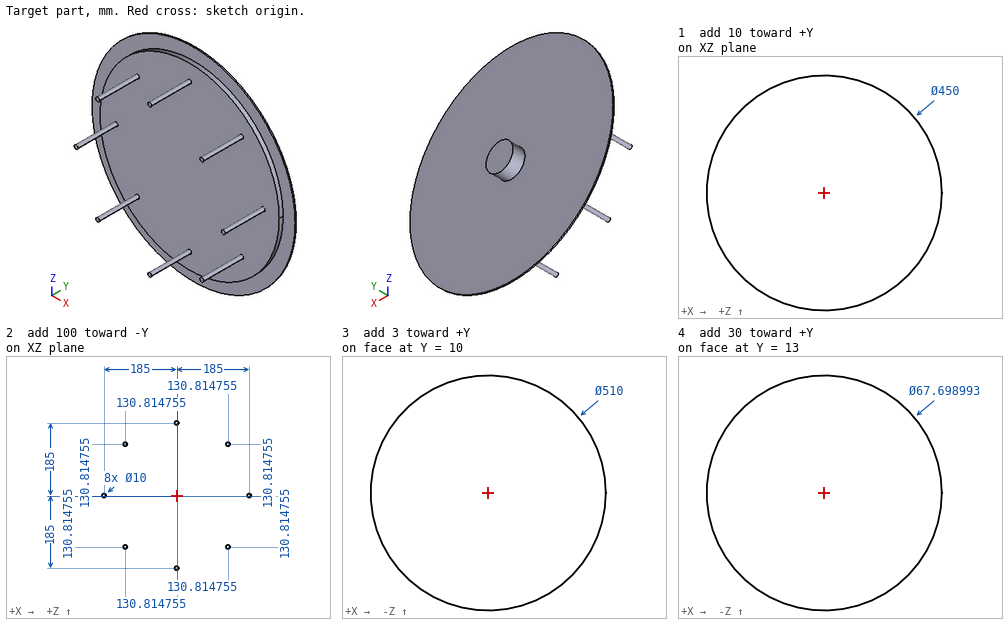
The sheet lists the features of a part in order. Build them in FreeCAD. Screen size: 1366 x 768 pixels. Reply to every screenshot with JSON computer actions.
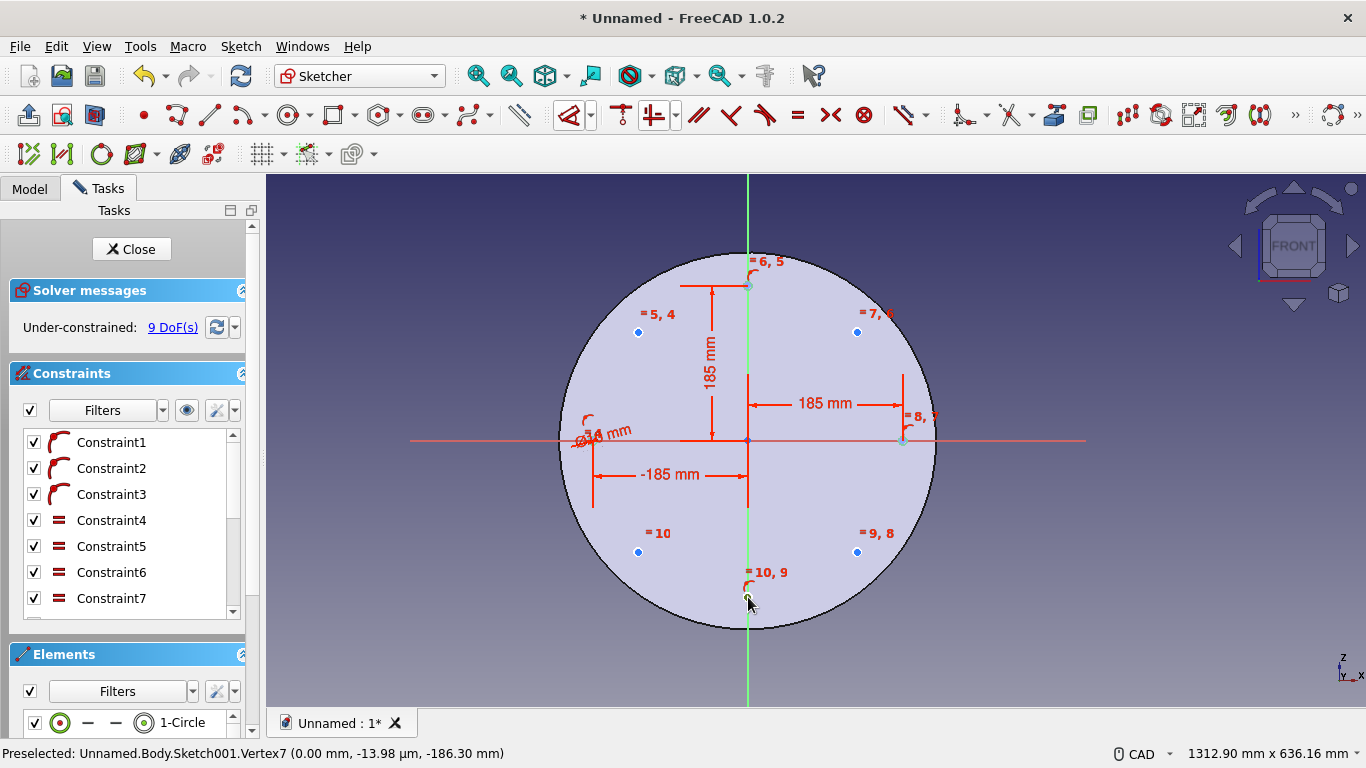
{"action": "key", "text": "i"}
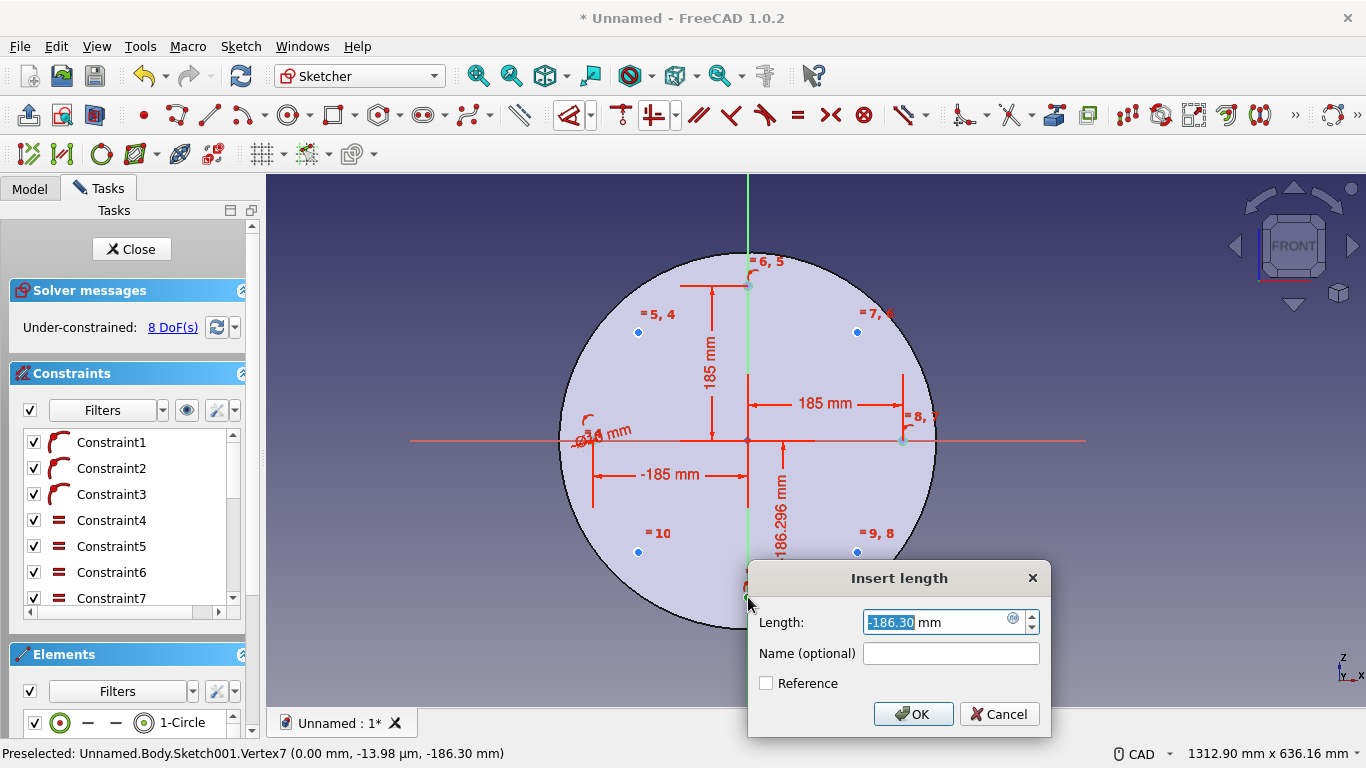
{"action": "type", "text": "-185"}
{"action": "key", "text": "Return"}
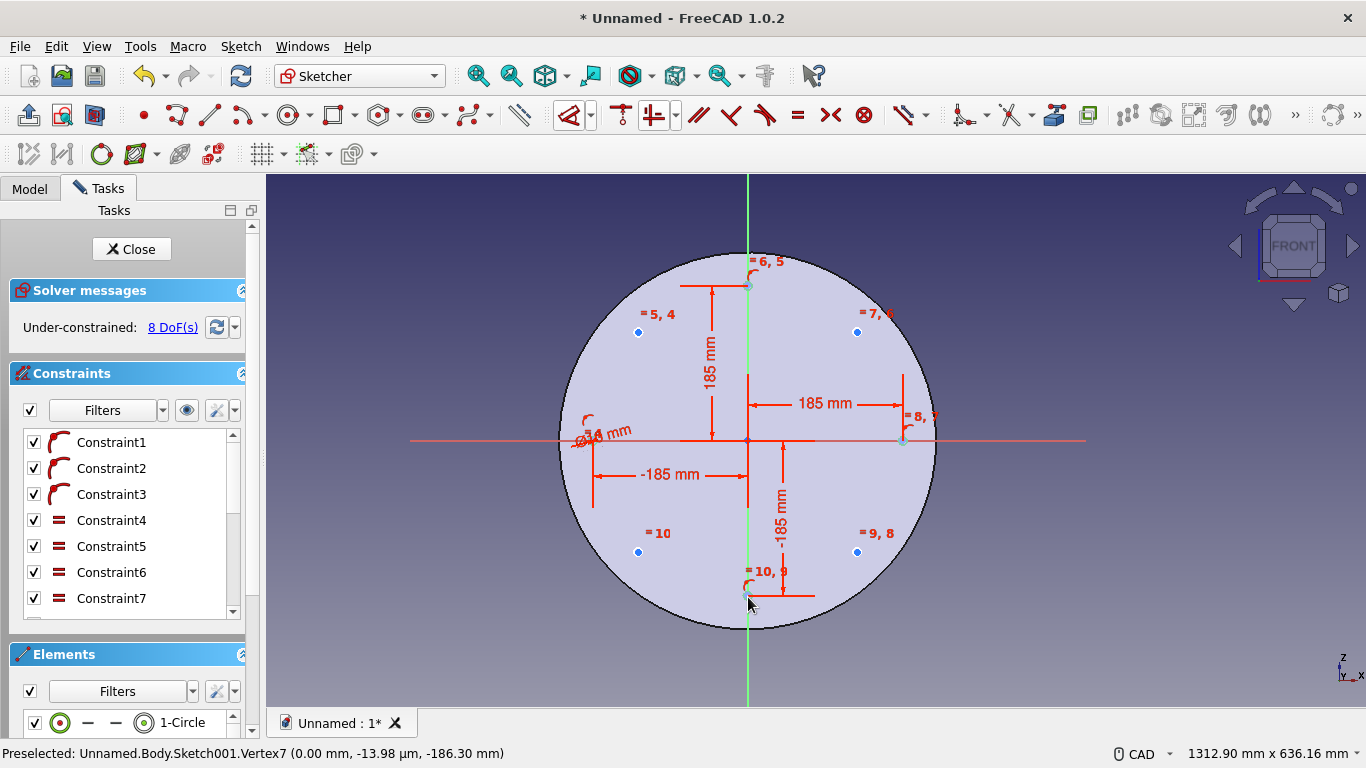
{"action": "left_click", "coordinate": [638, 333]}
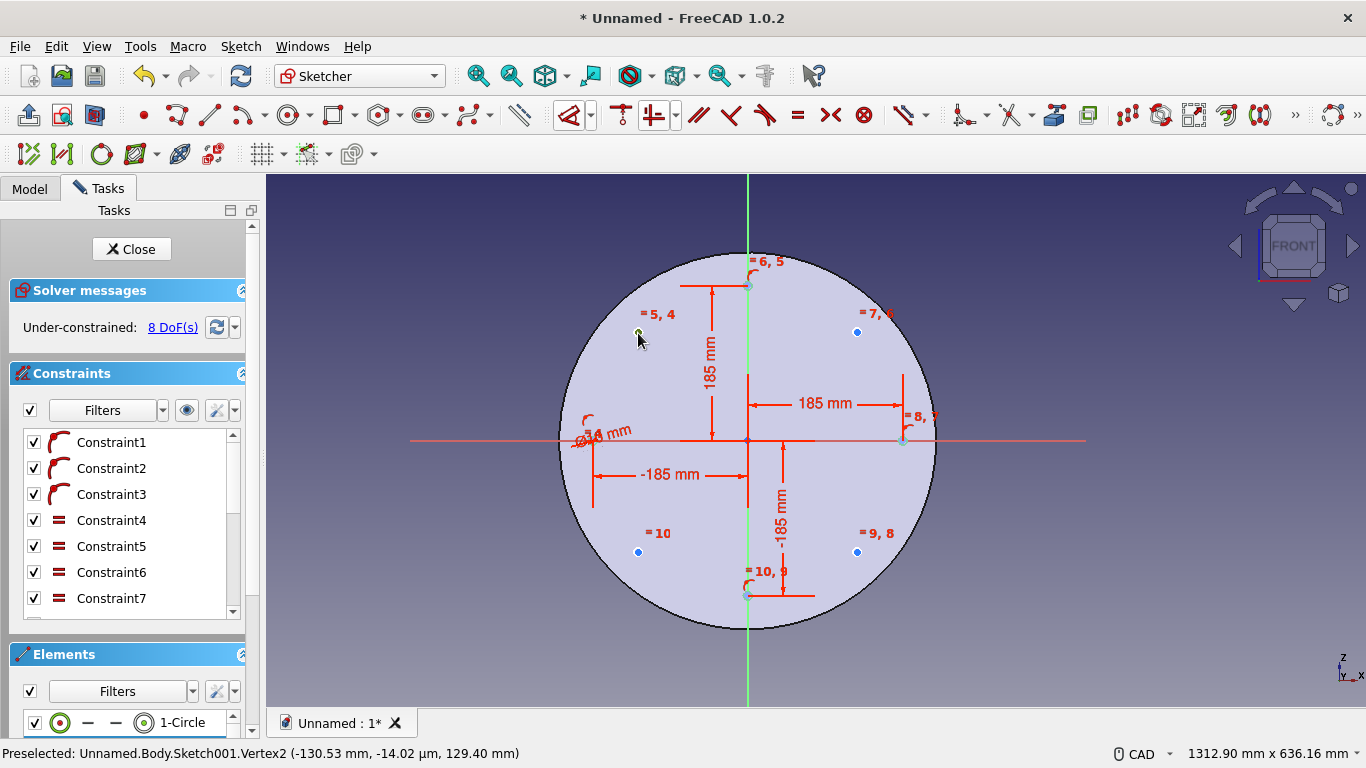
{"action": "key", "text": "l"}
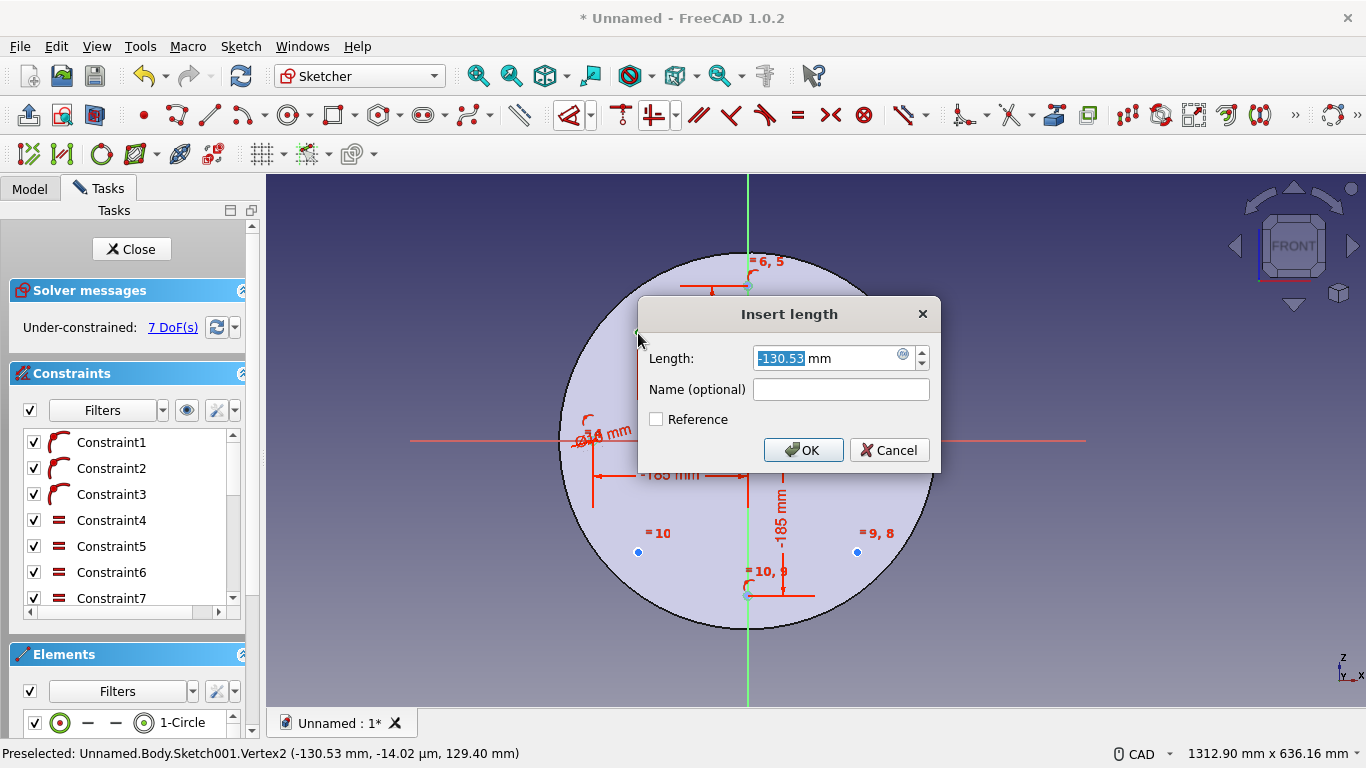
{"action": "type", "text": "-130.814755"}
{"action": "key", "text": "Return"}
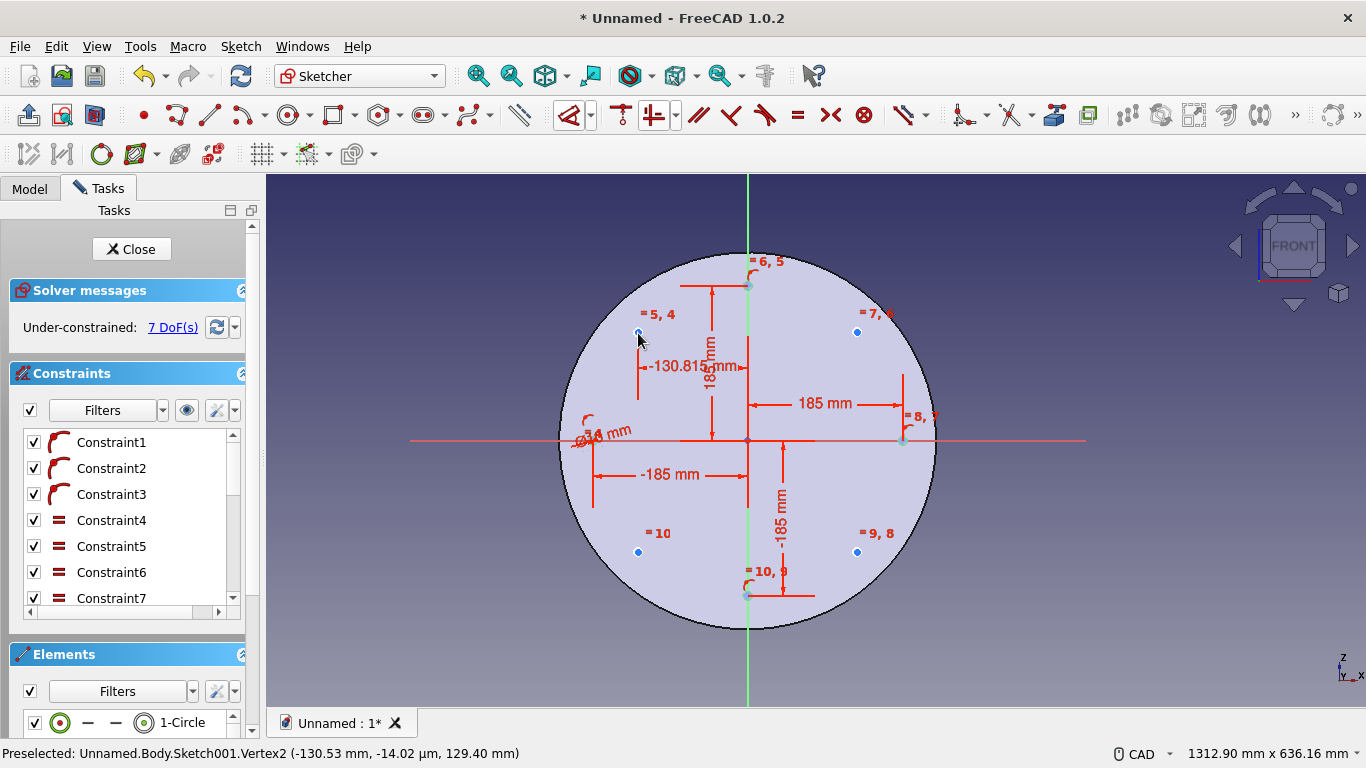
{"action": "left_click", "coordinate": [638, 333]}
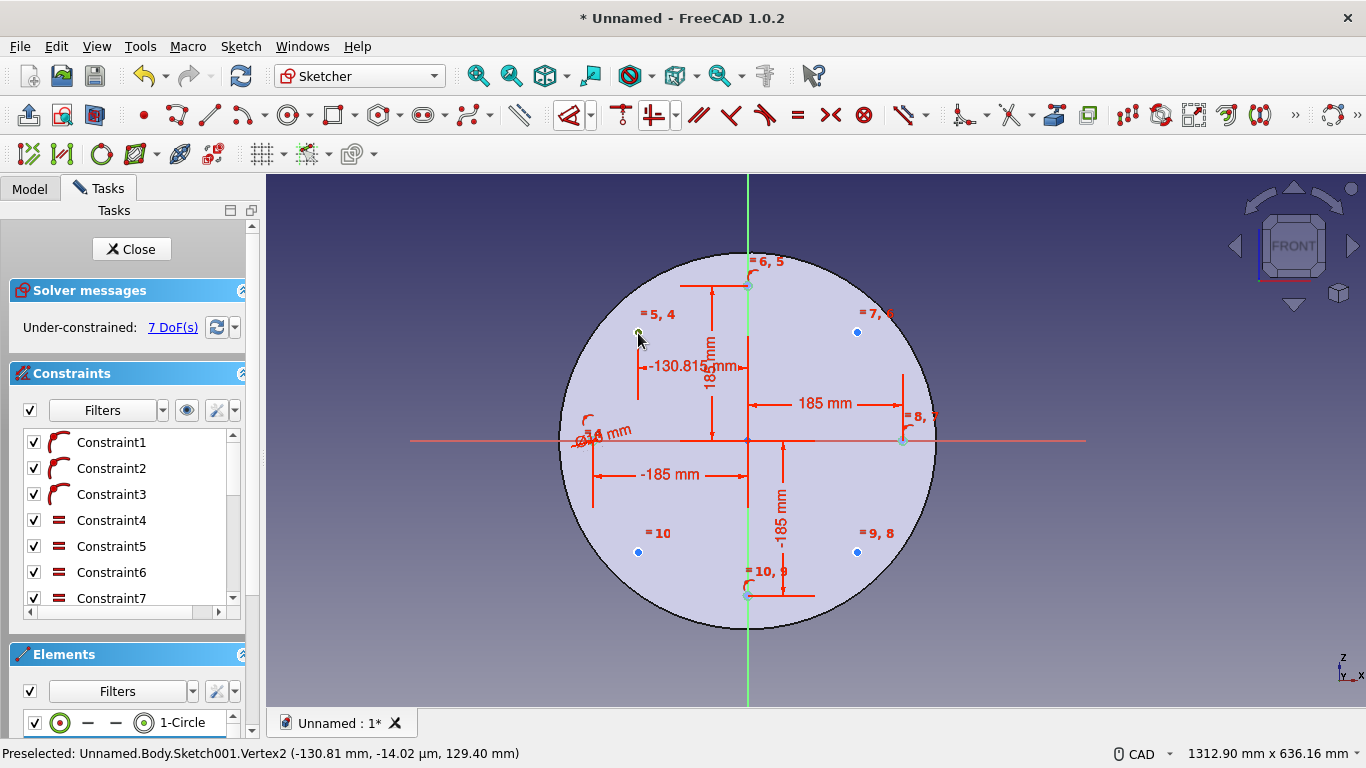
{"action": "key", "text": "i"}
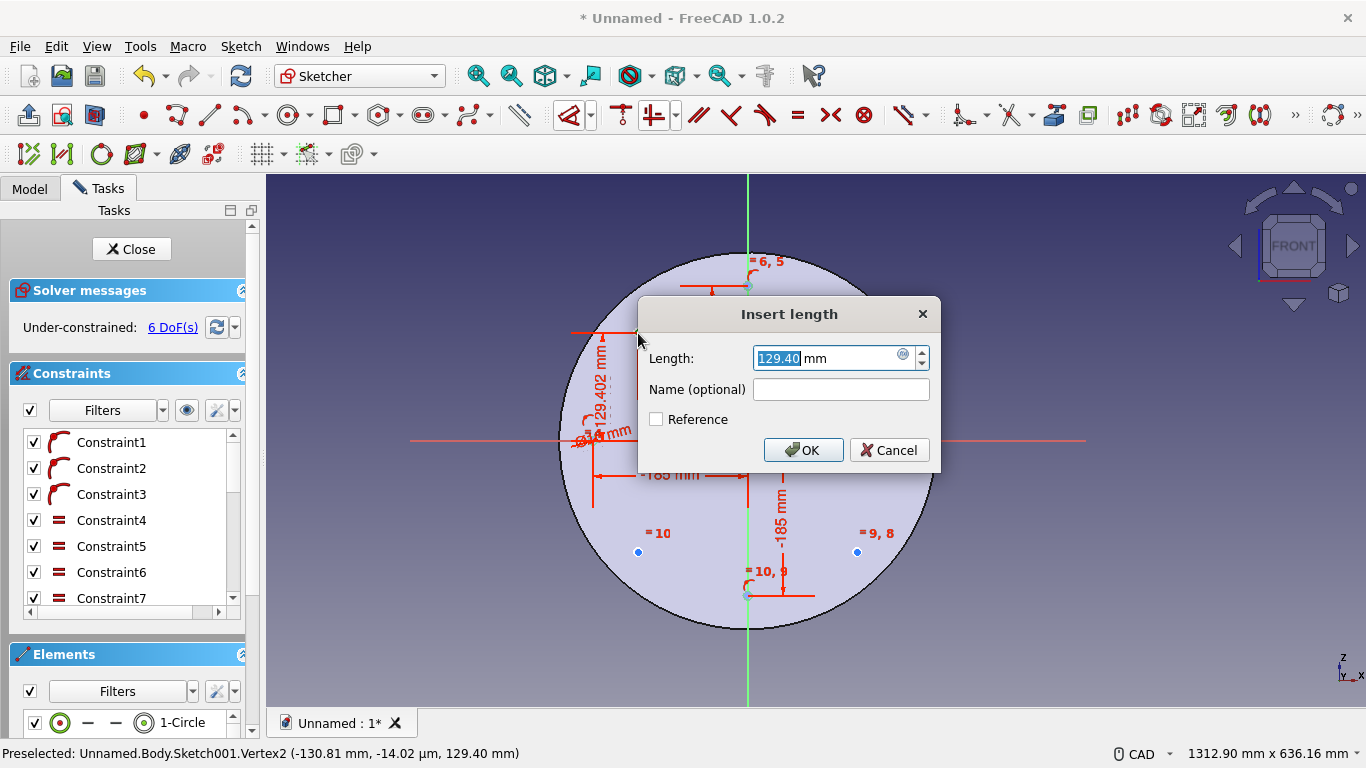
{"action": "type", "text": "130.814755"}
{"action": "key", "text": "Return"}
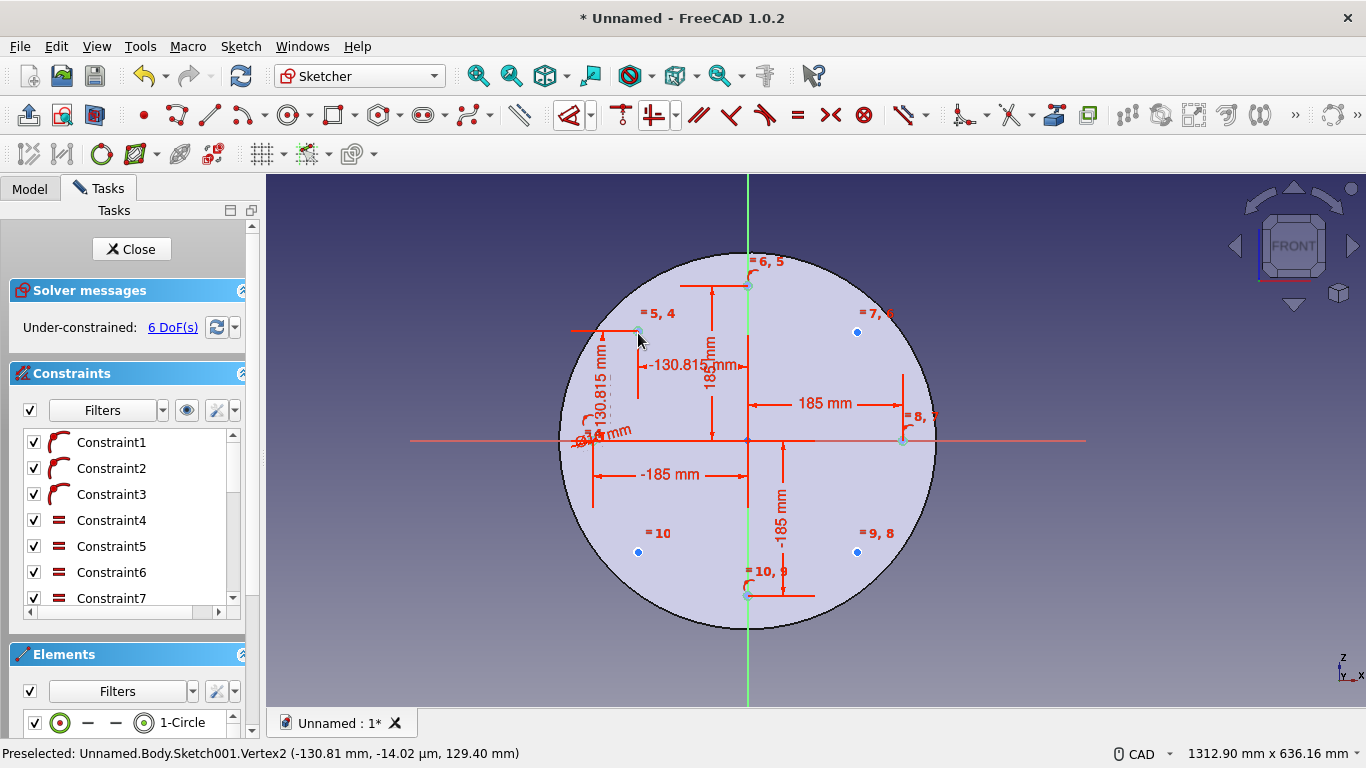
{"action": "left_click", "coordinate": [857, 332]}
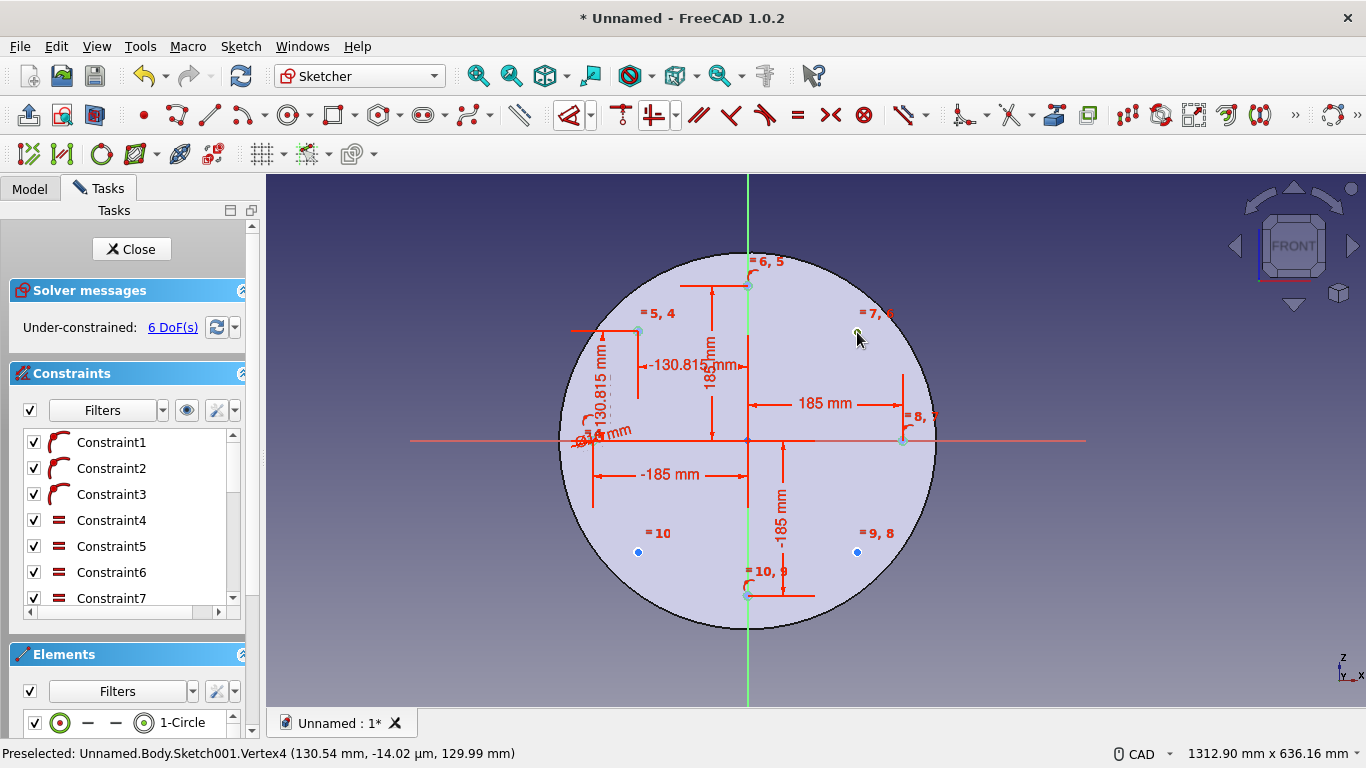
{"action": "left_click", "coordinate": [590, 116]}